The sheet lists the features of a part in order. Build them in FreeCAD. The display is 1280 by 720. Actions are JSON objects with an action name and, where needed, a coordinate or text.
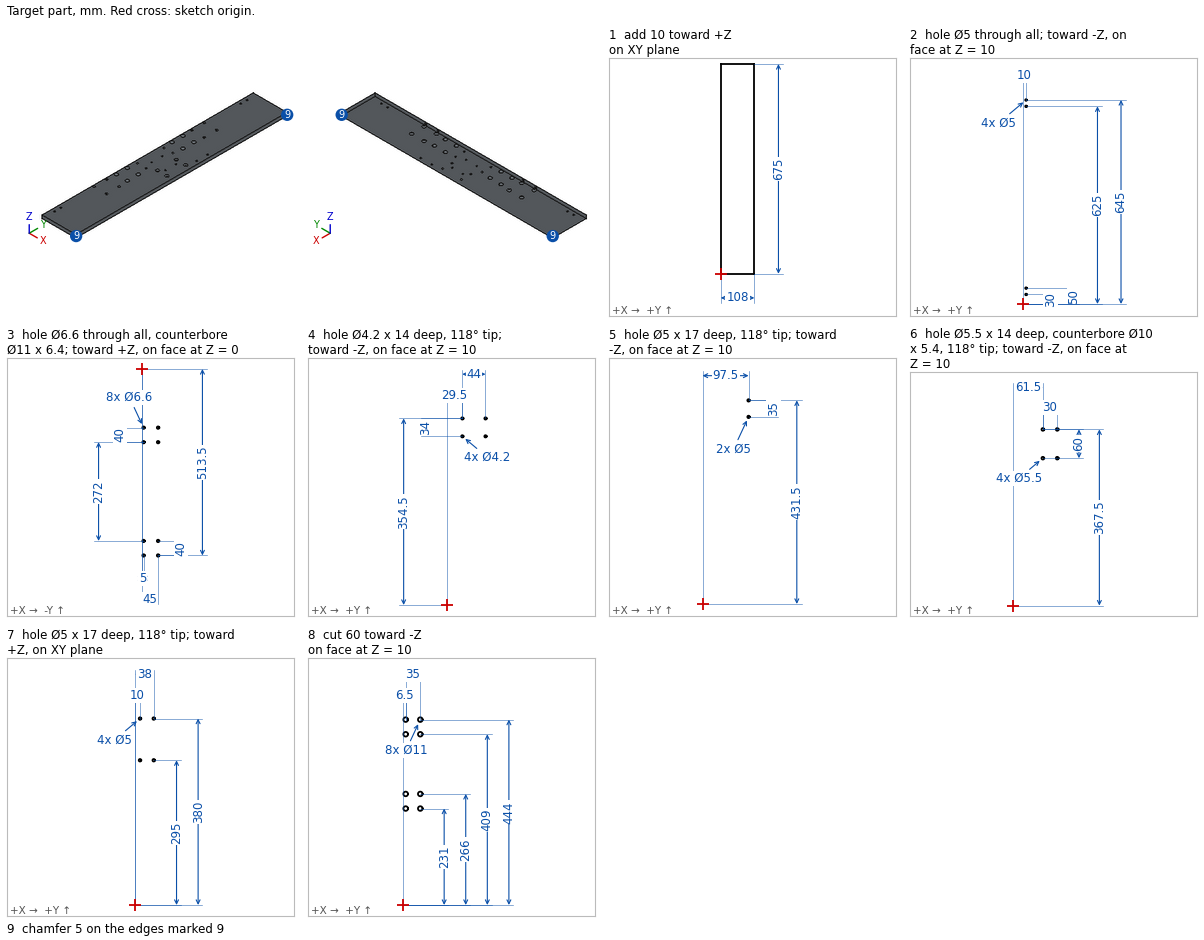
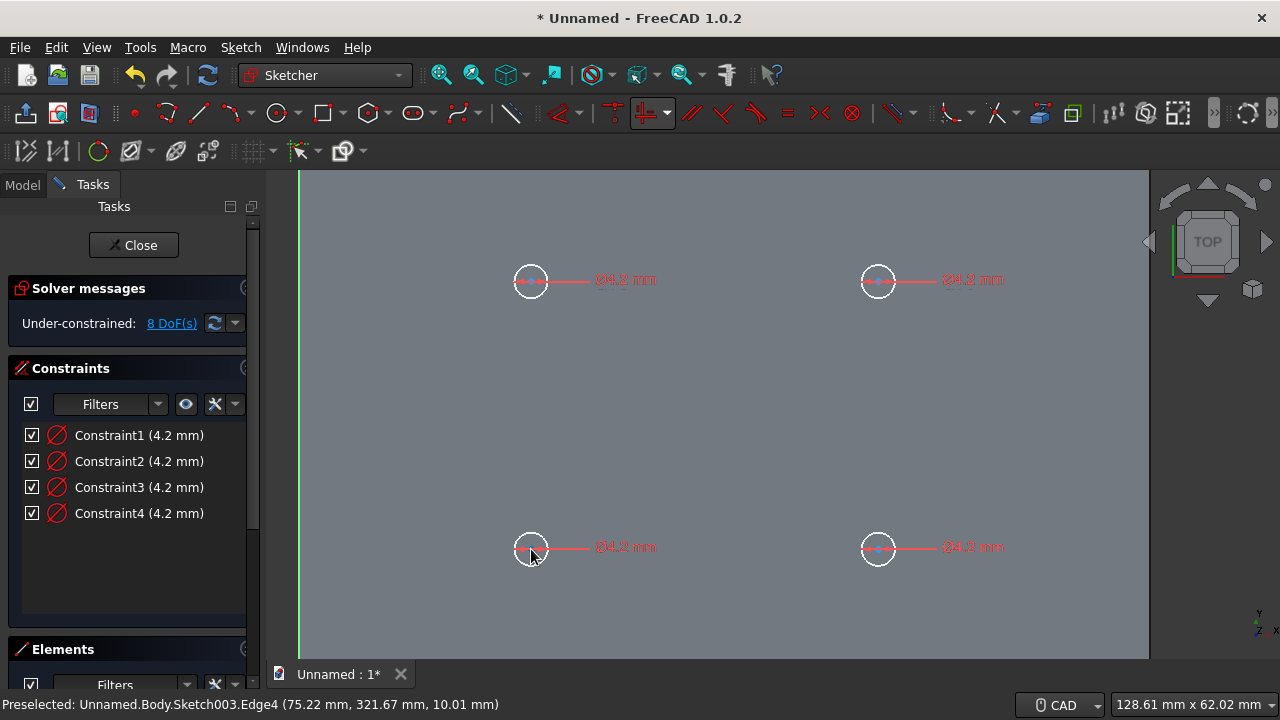
{"action": "left_click", "coordinate": [531, 282]}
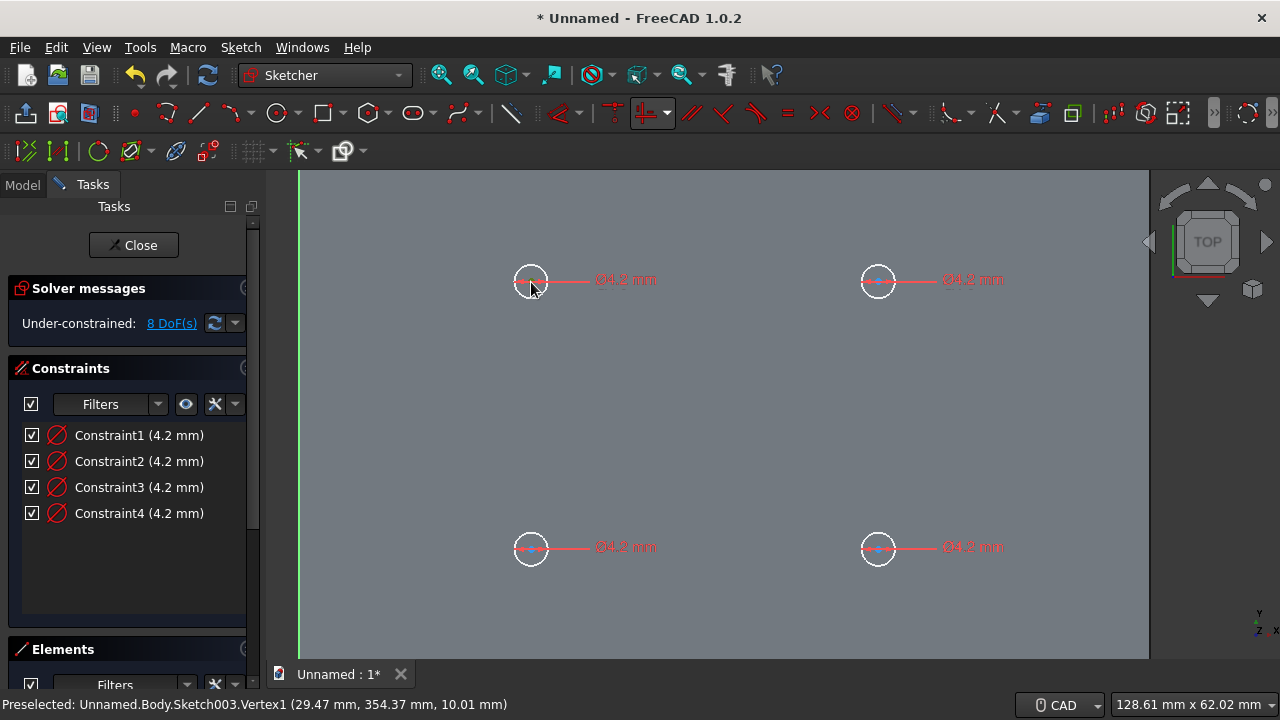
{"action": "left_click", "coordinate": [878, 282]}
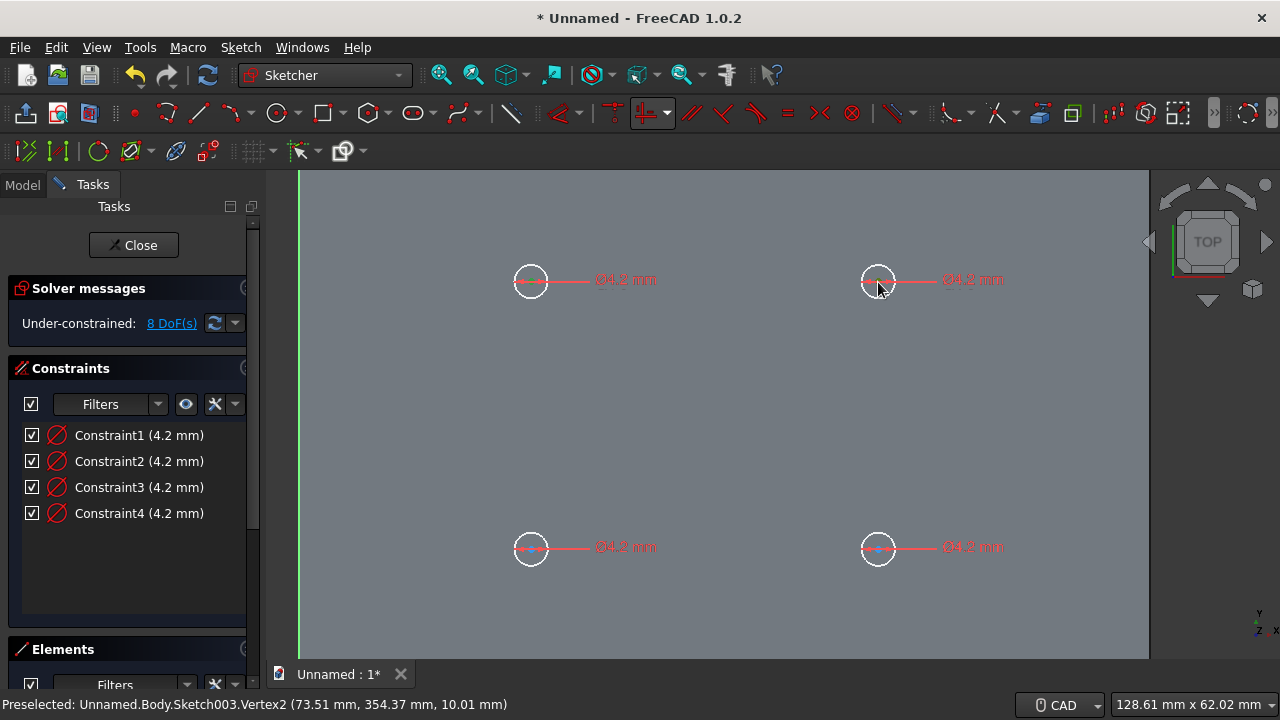
{"action": "left_click", "coordinate": [670, 114]}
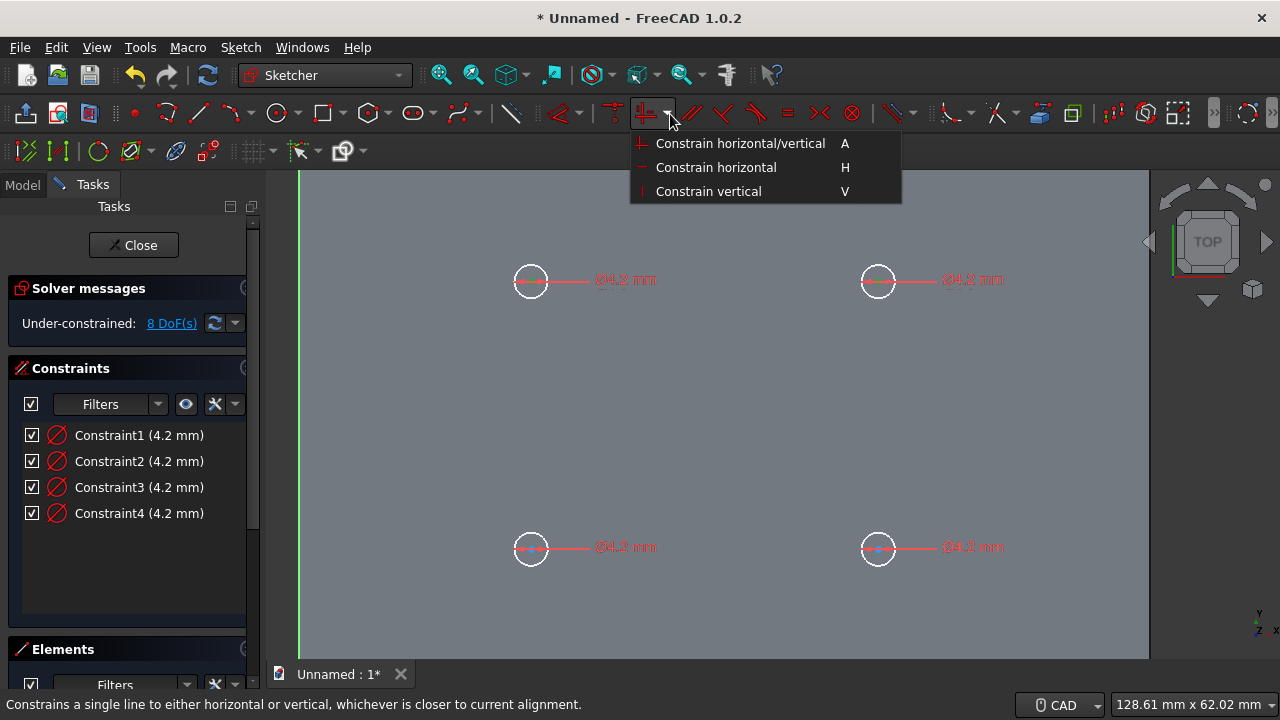
{"action": "left_click", "coordinate": [766, 167]}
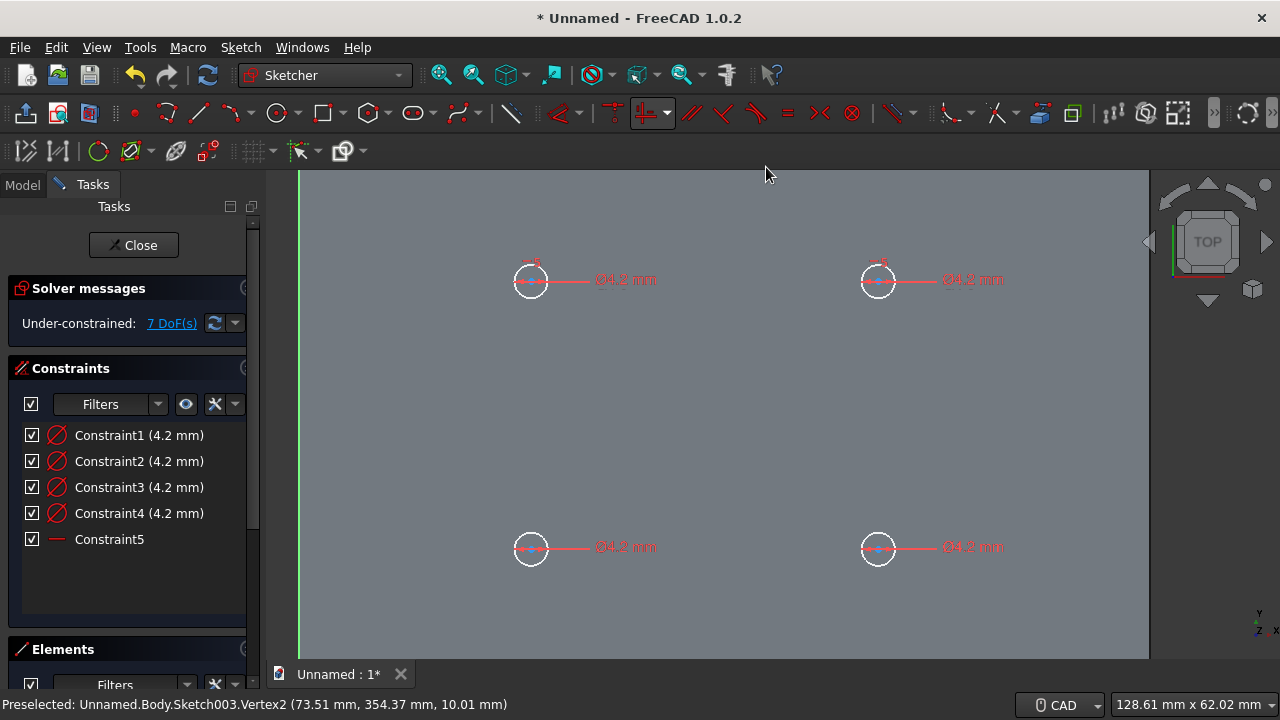
{"action": "left_click", "coordinate": [531, 282]}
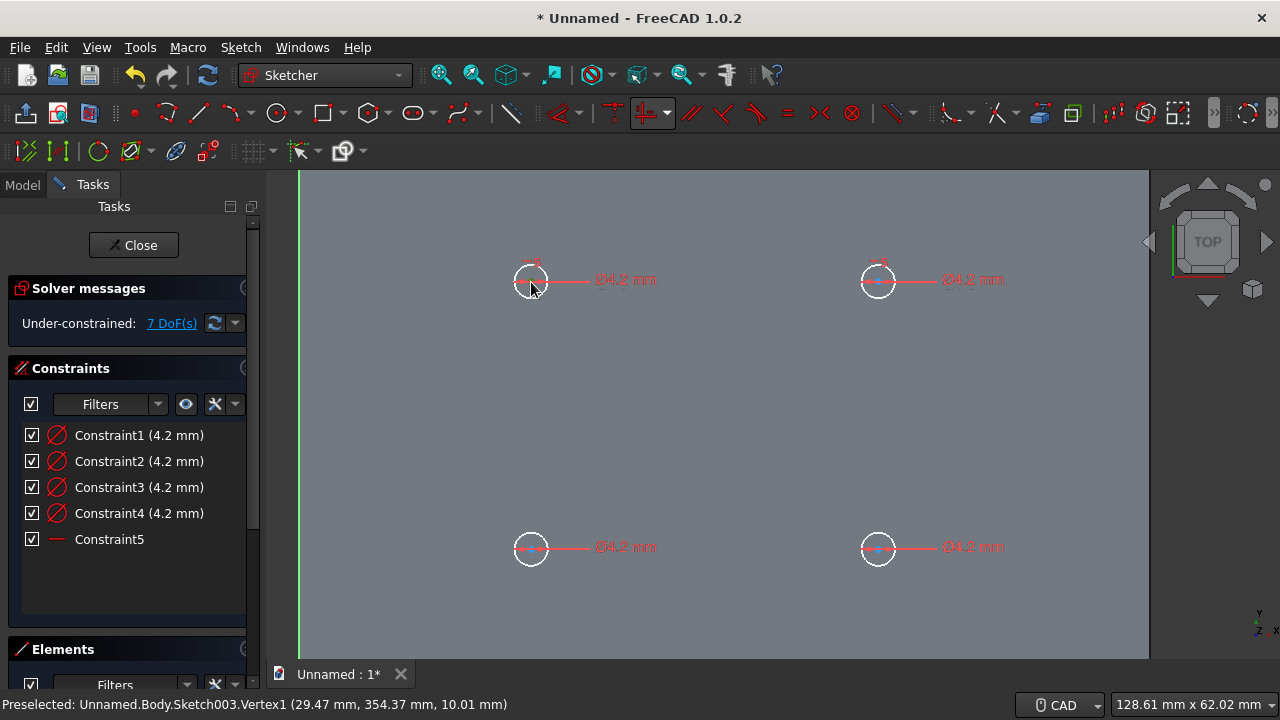
{"action": "left_click", "coordinate": [531, 549]}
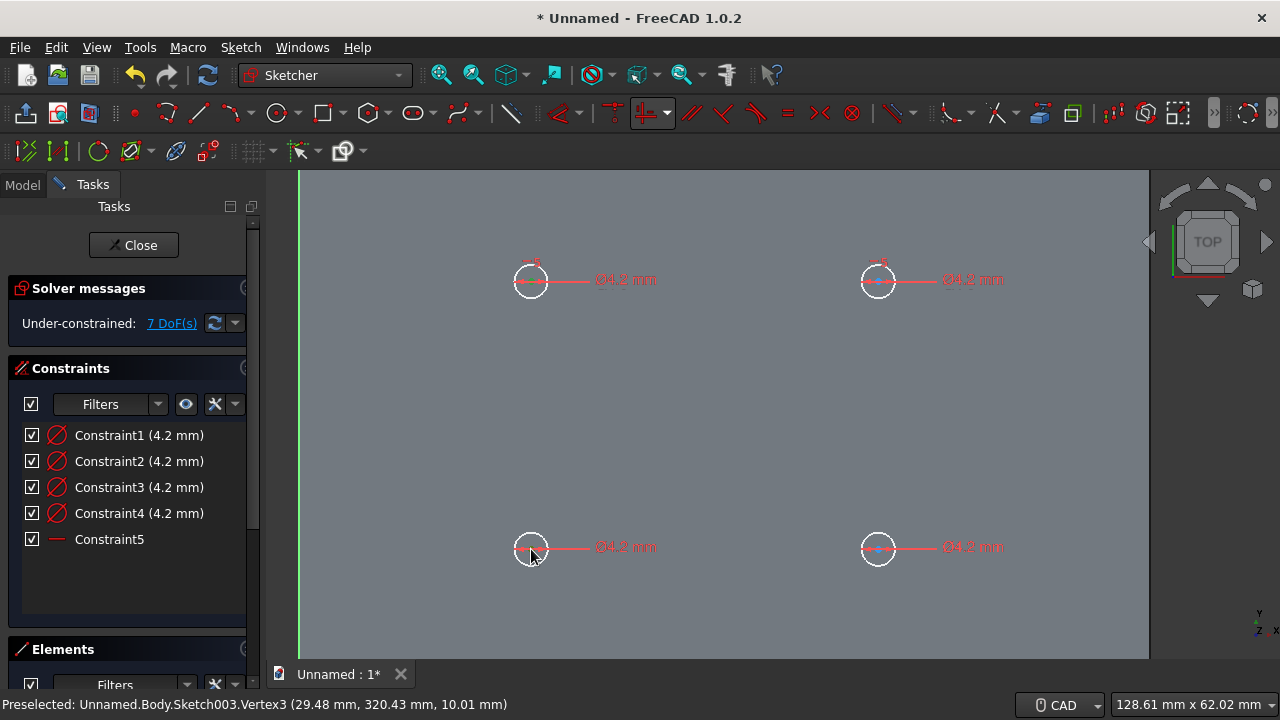
{"action": "key", "text": "v"}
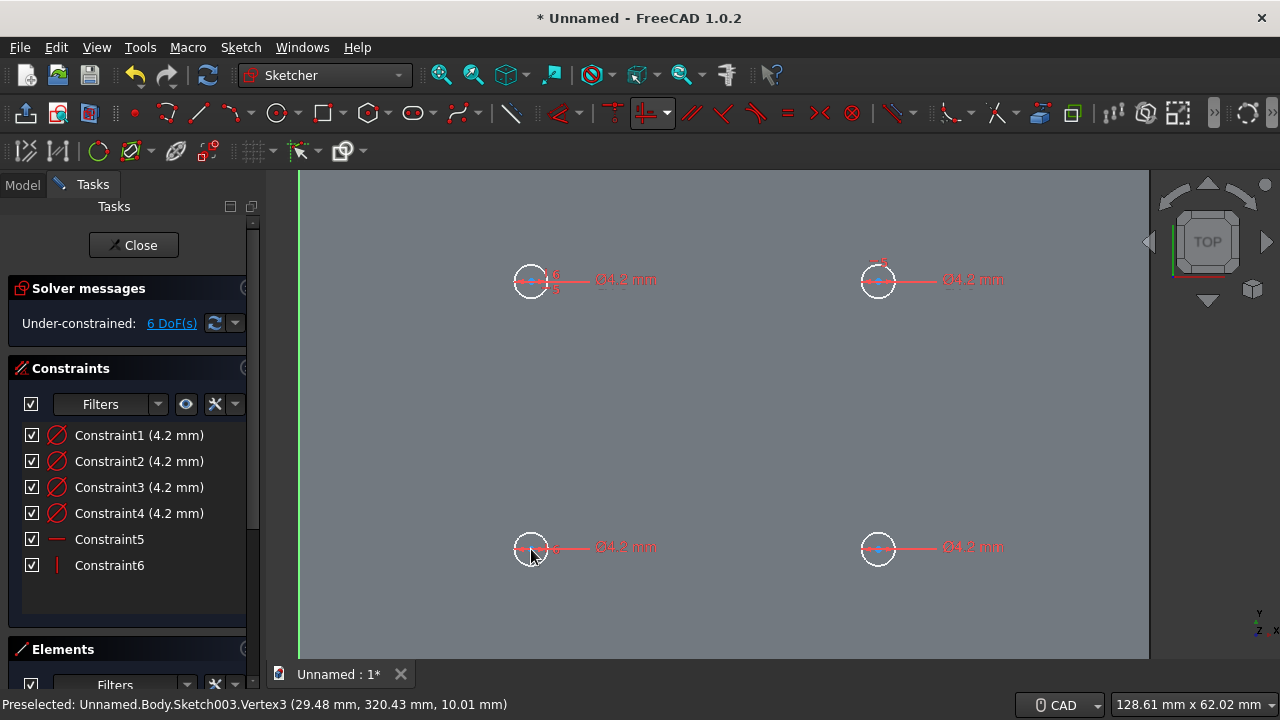
{"action": "left_click", "coordinate": [878, 282]}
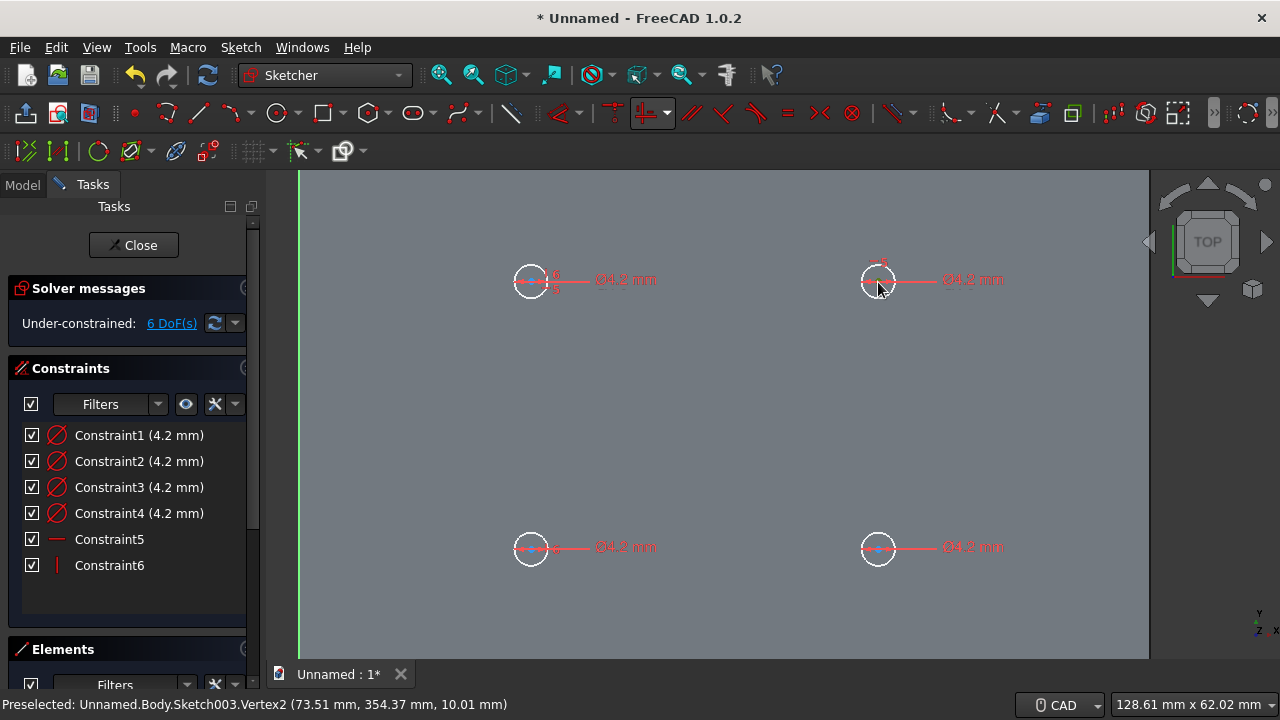
{"action": "left_click", "coordinate": [878, 549]}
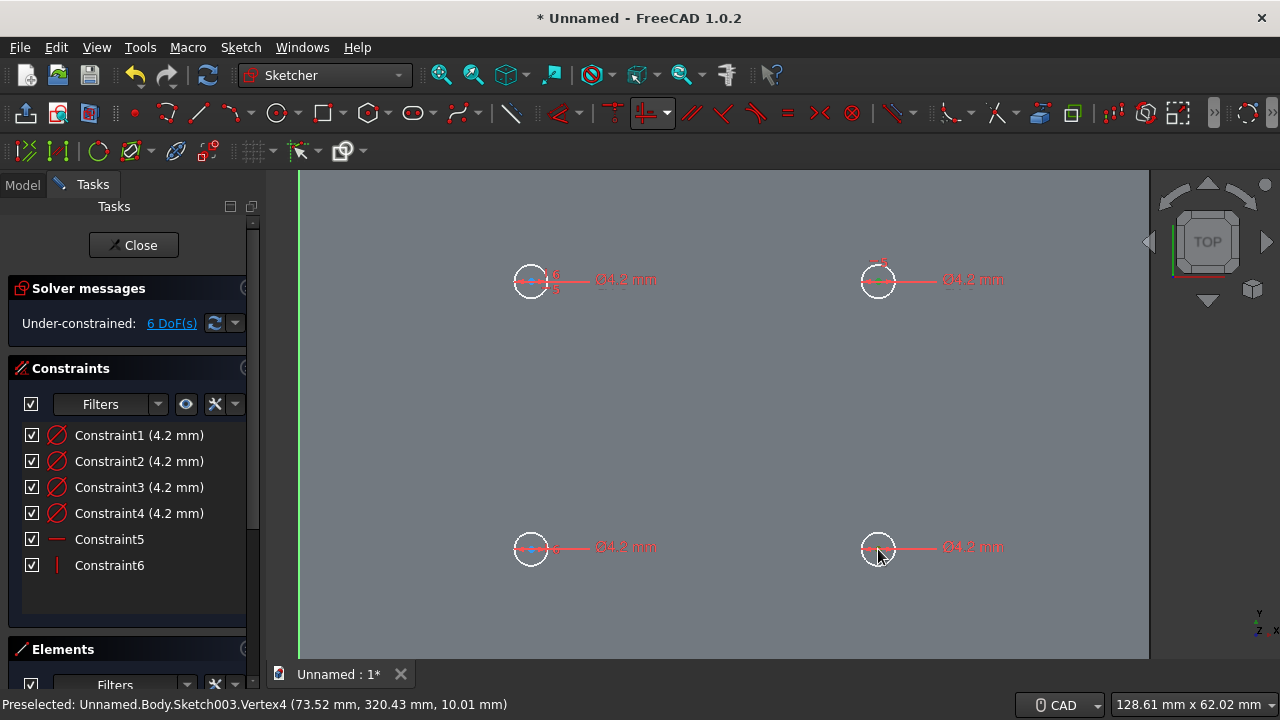
{"action": "left_click", "coordinate": [670, 114]}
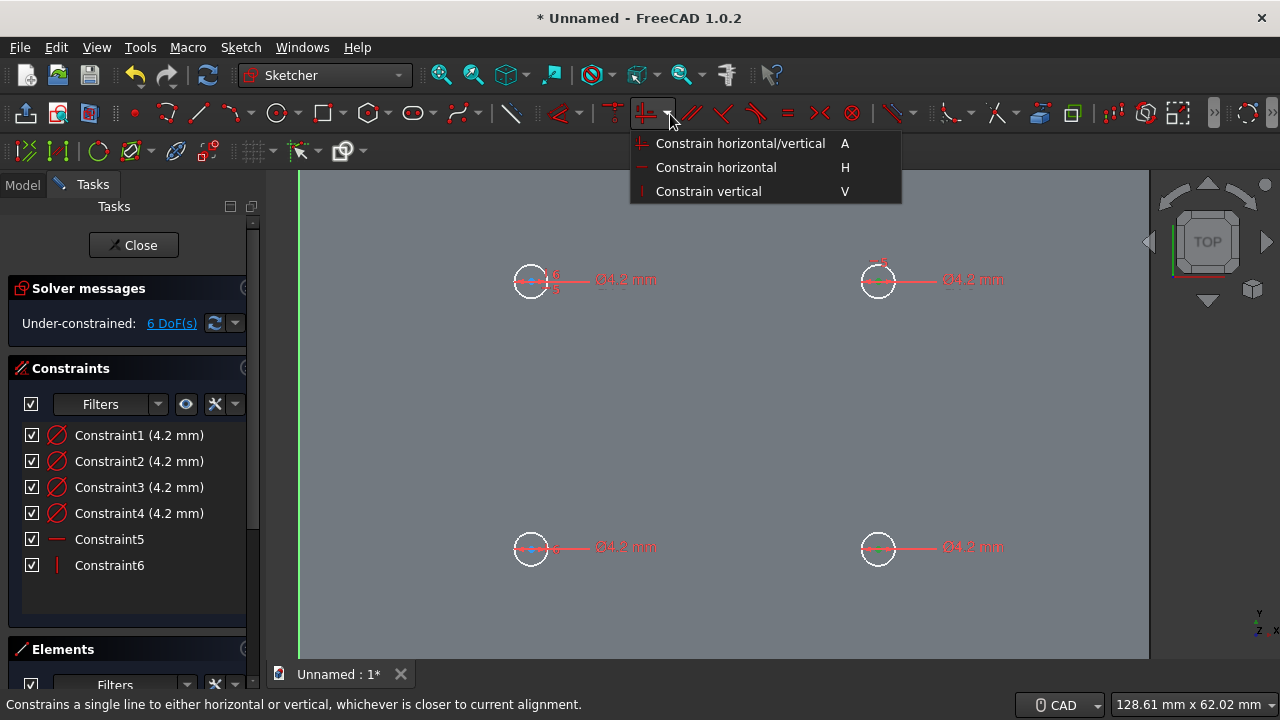
{"action": "left_click", "coordinate": [766, 191]}